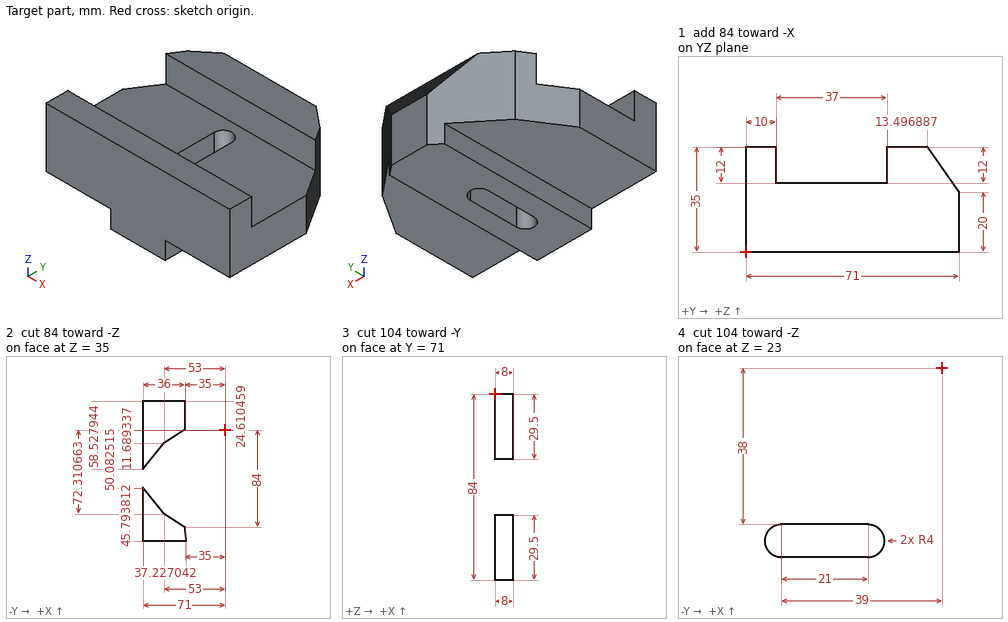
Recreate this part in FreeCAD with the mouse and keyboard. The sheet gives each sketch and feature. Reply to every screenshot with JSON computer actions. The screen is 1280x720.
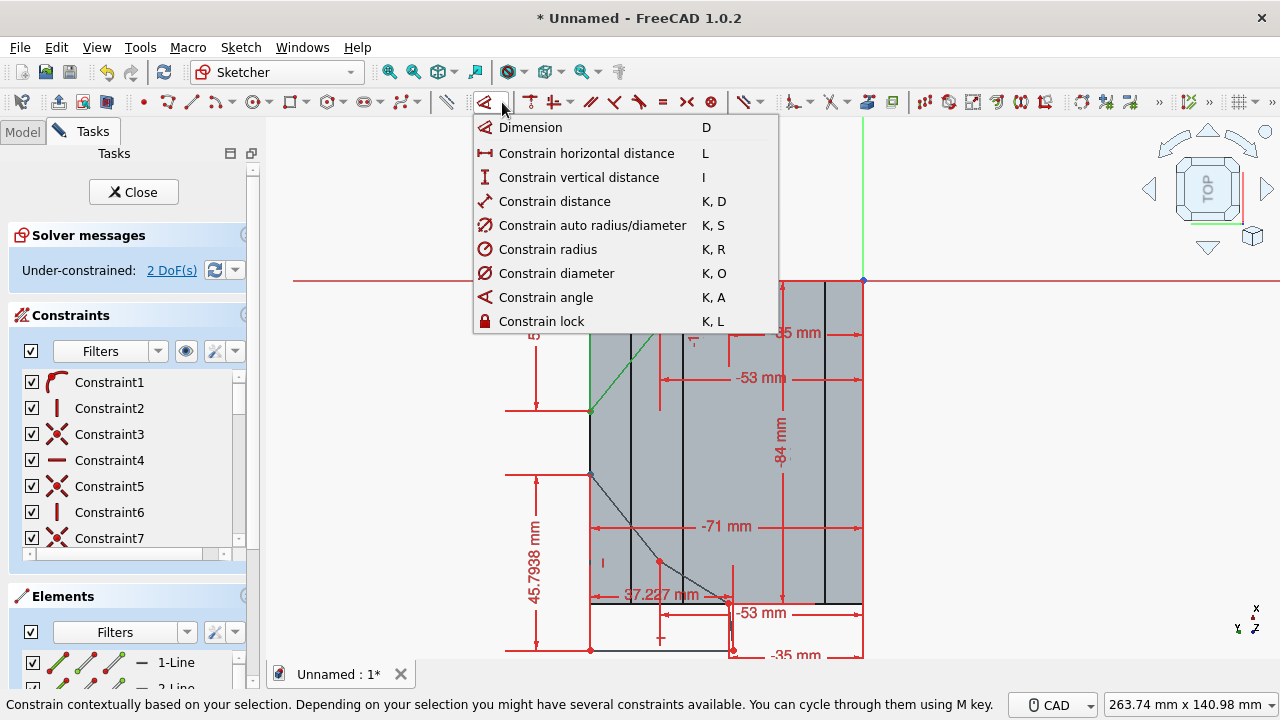
{"action": "left_click", "coordinate": [626, 177]}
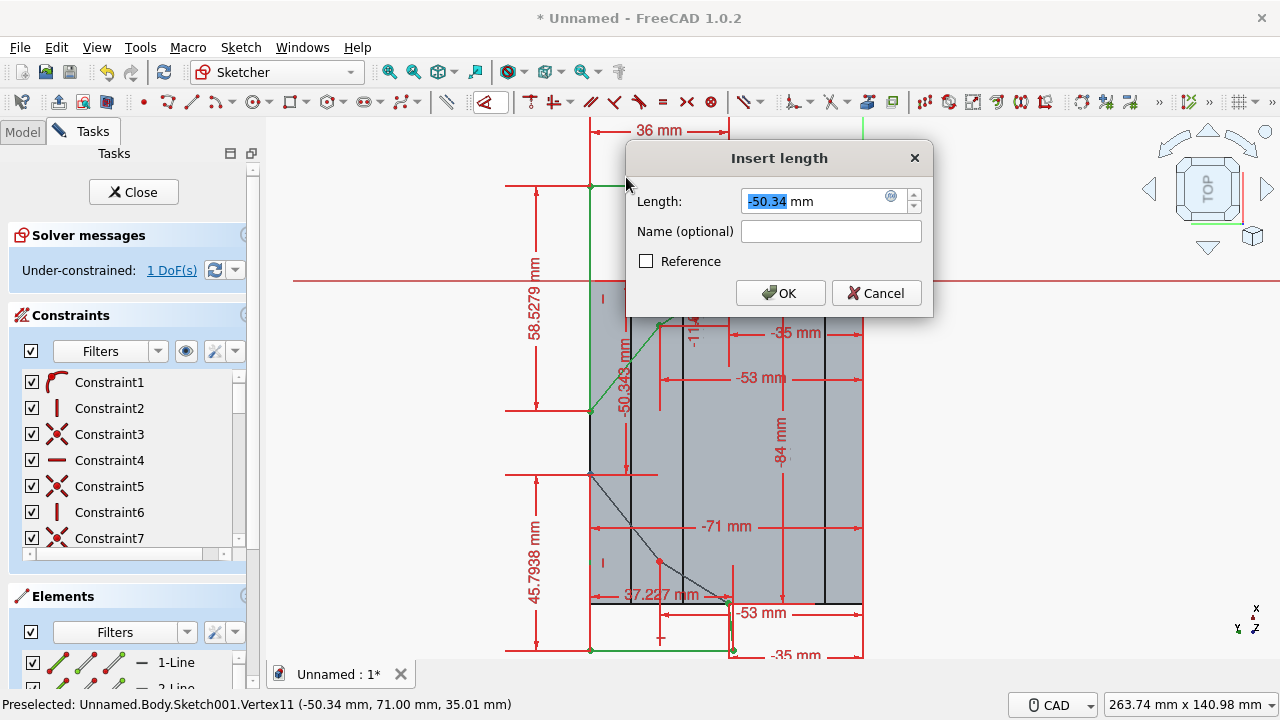
{"action": "type", "text": "-50.082515"}
{"action": "key", "text": "Return"}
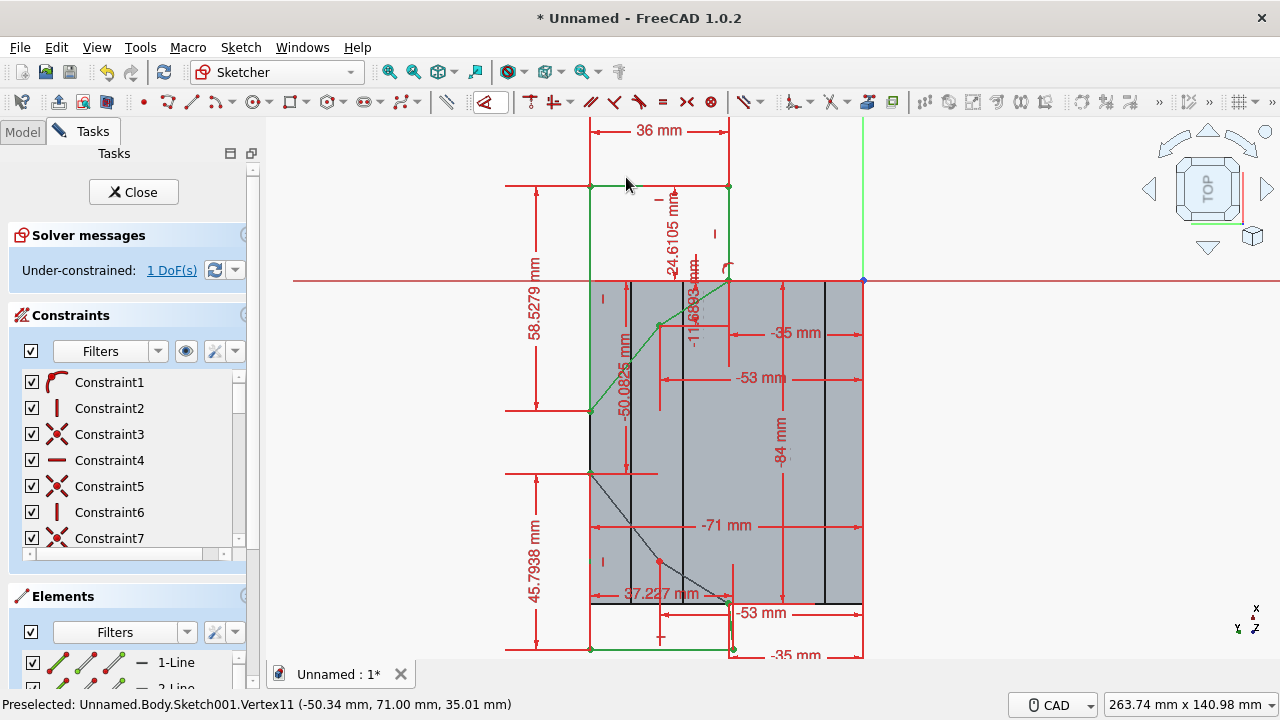
{"action": "left_click", "coordinate": [660, 561]}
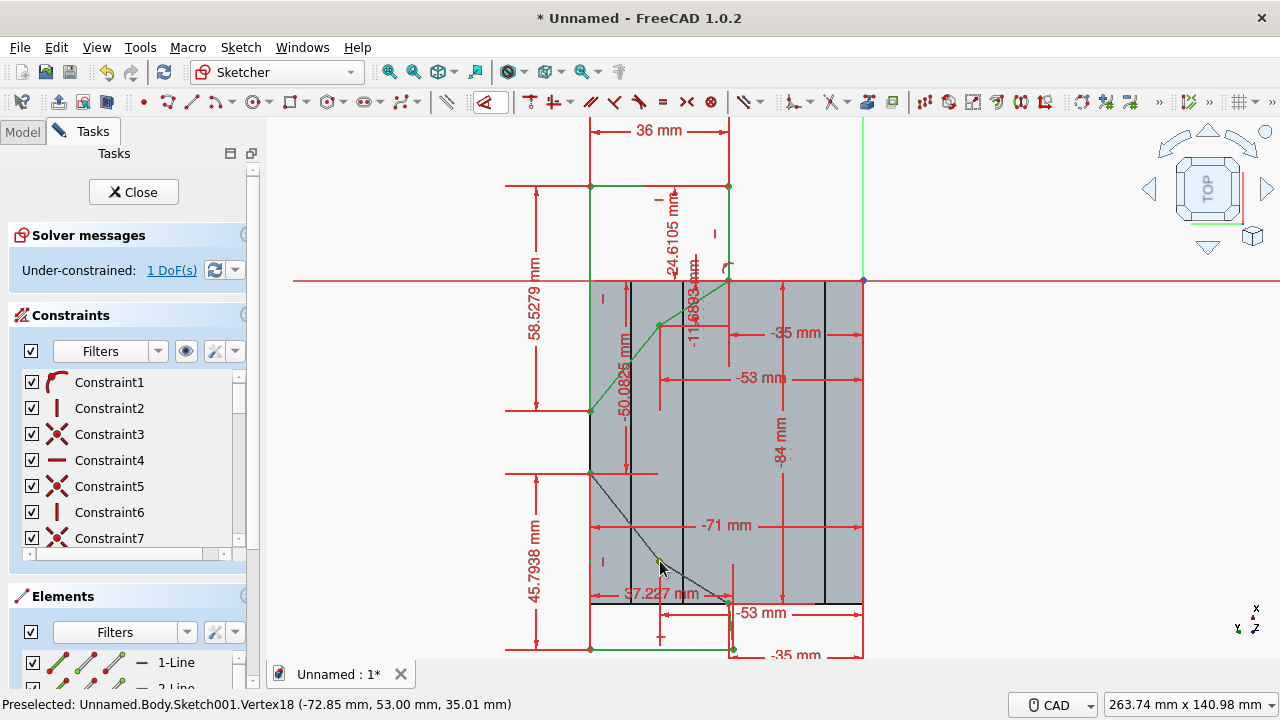
{"action": "left_click", "coordinate": [502, 102]}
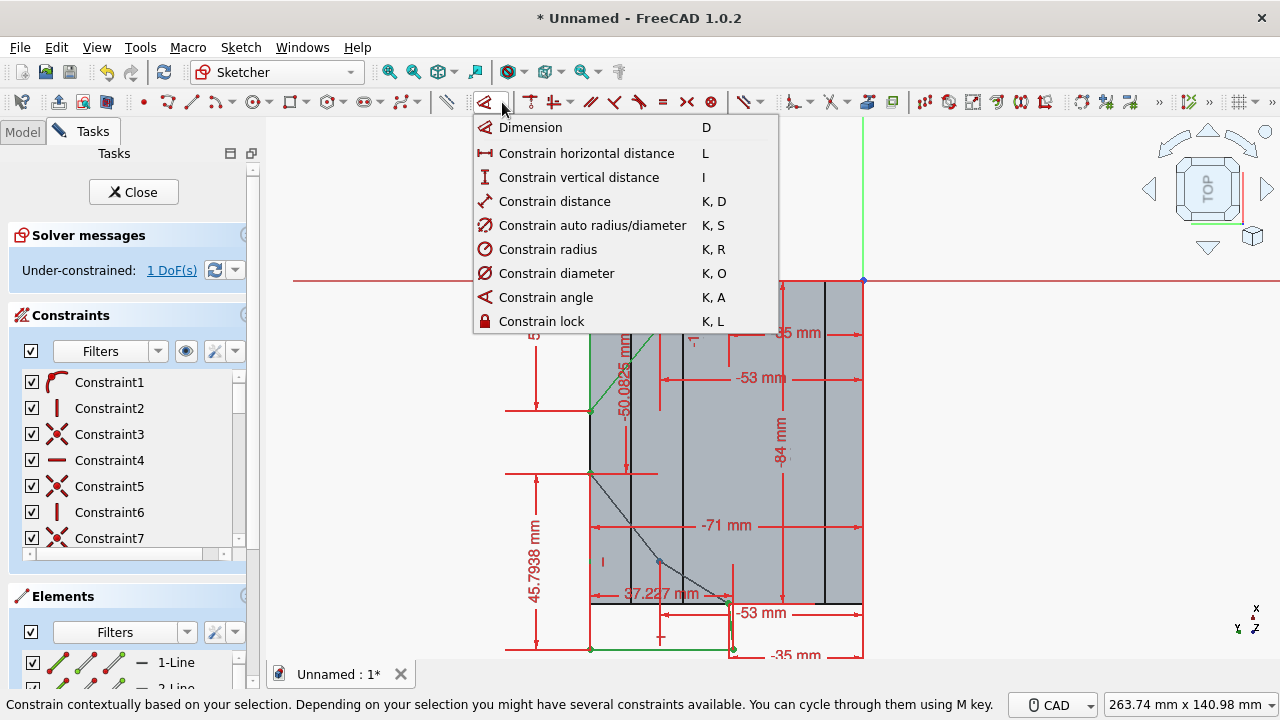
{"action": "left_click", "coordinate": [626, 177]}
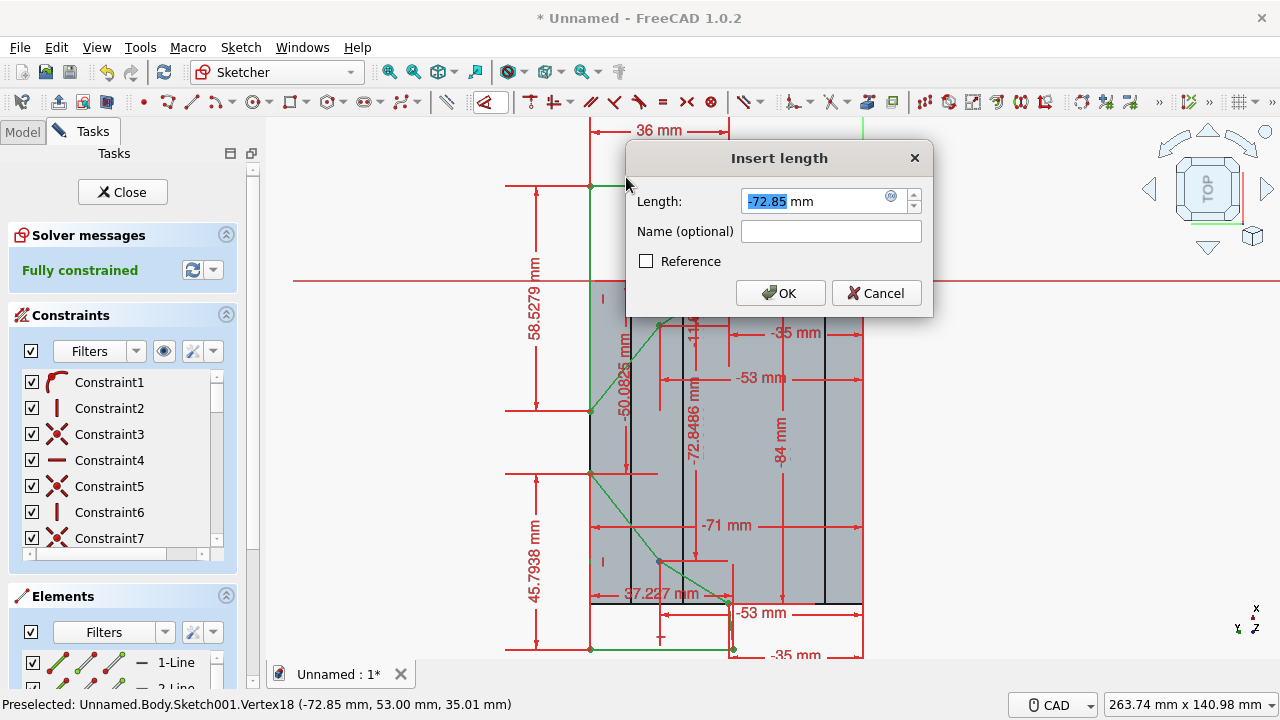
{"action": "type", "text": "-72.310663"}
{"action": "key", "text": "Return"}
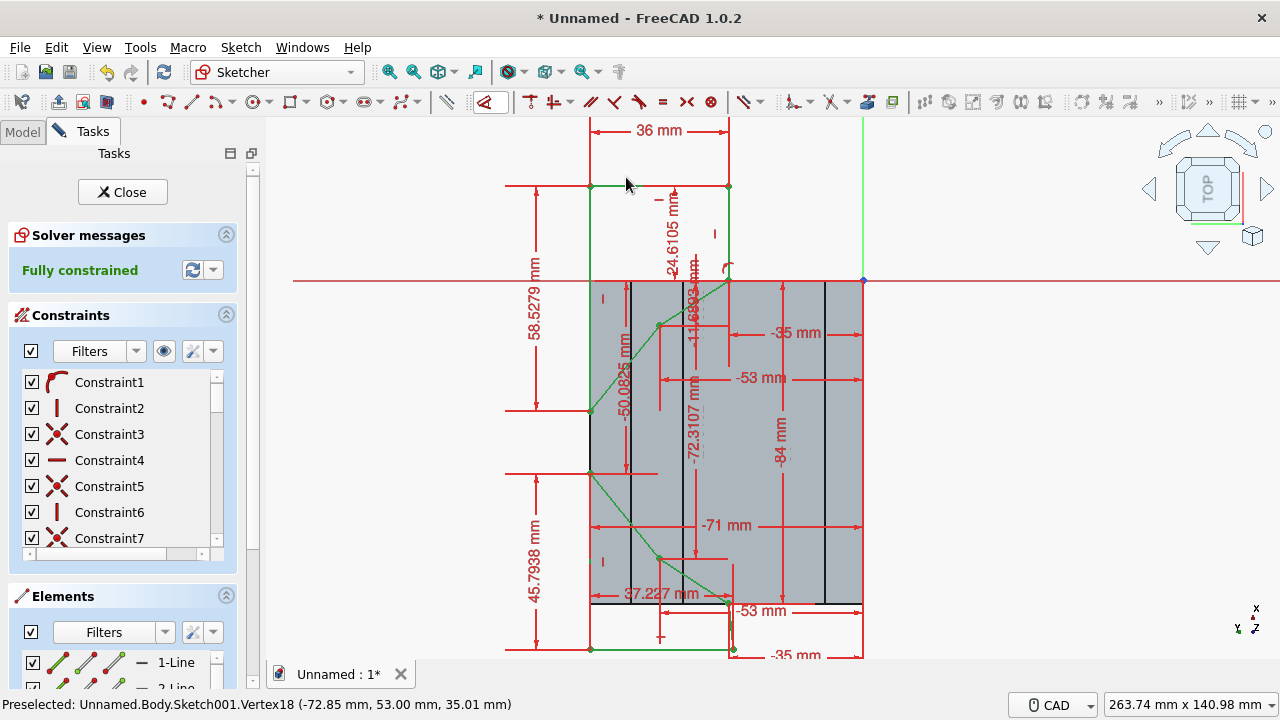
{"action": "left_click", "coordinate": [123, 192]}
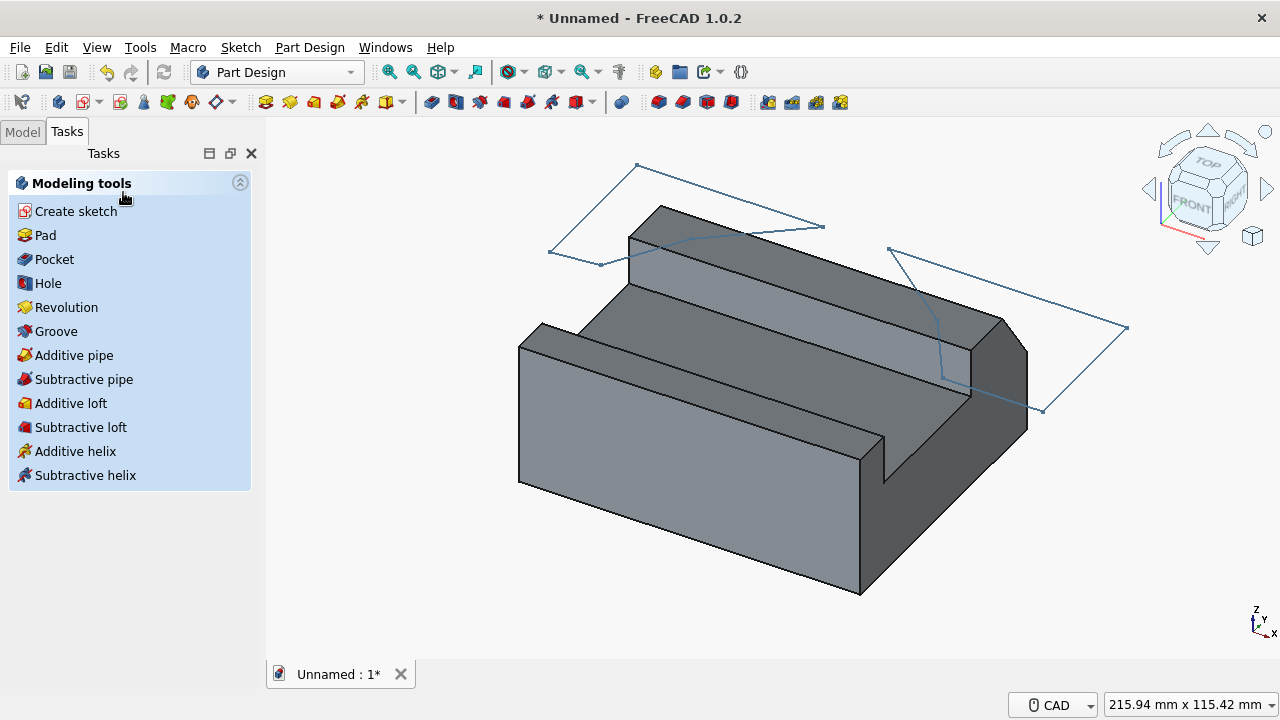
{"action": "left_click", "coordinate": [432, 102]}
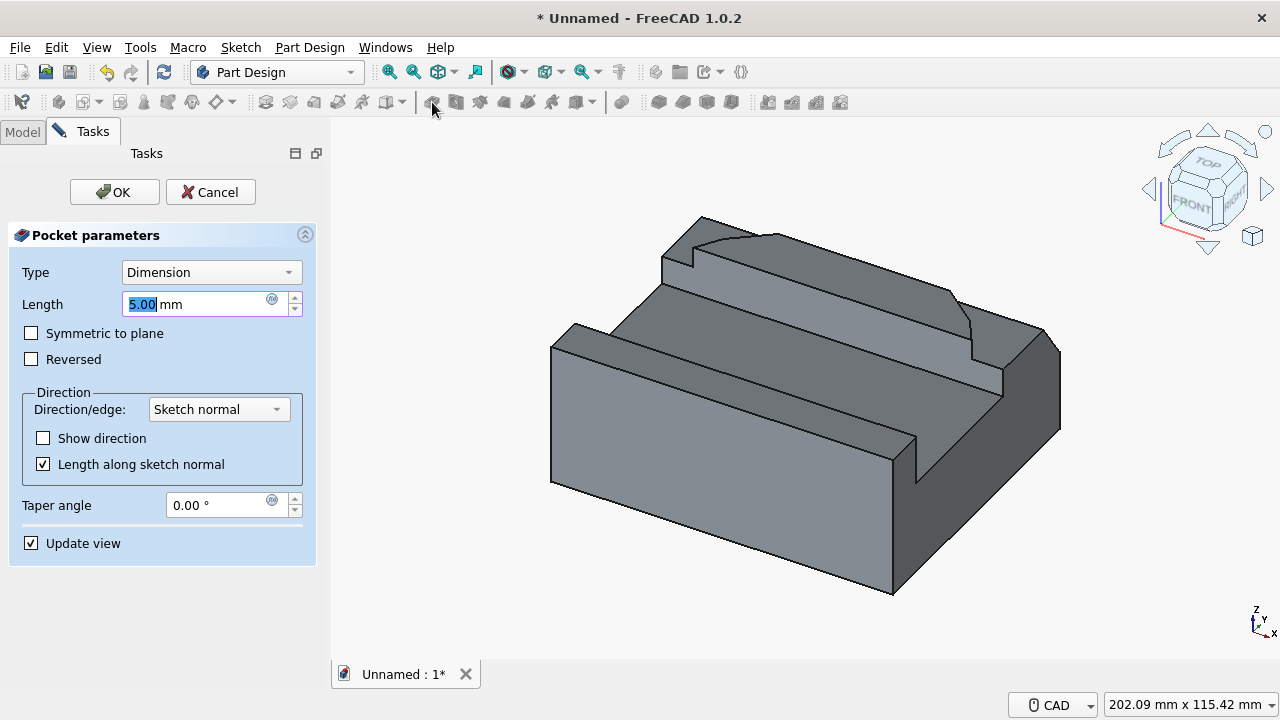
{"action": "type", "text": "84"}
{"action": "key", "text": "Tab"}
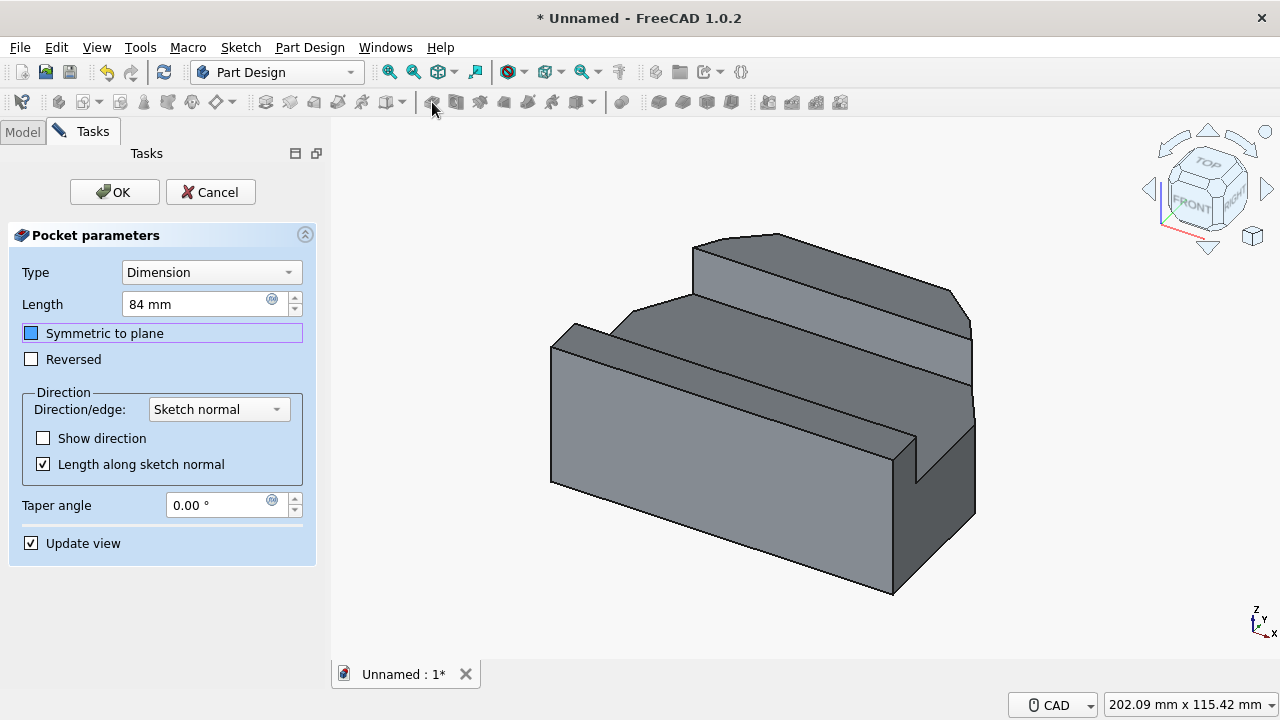
{"action": "left_click", "coordinate": [115, 192]}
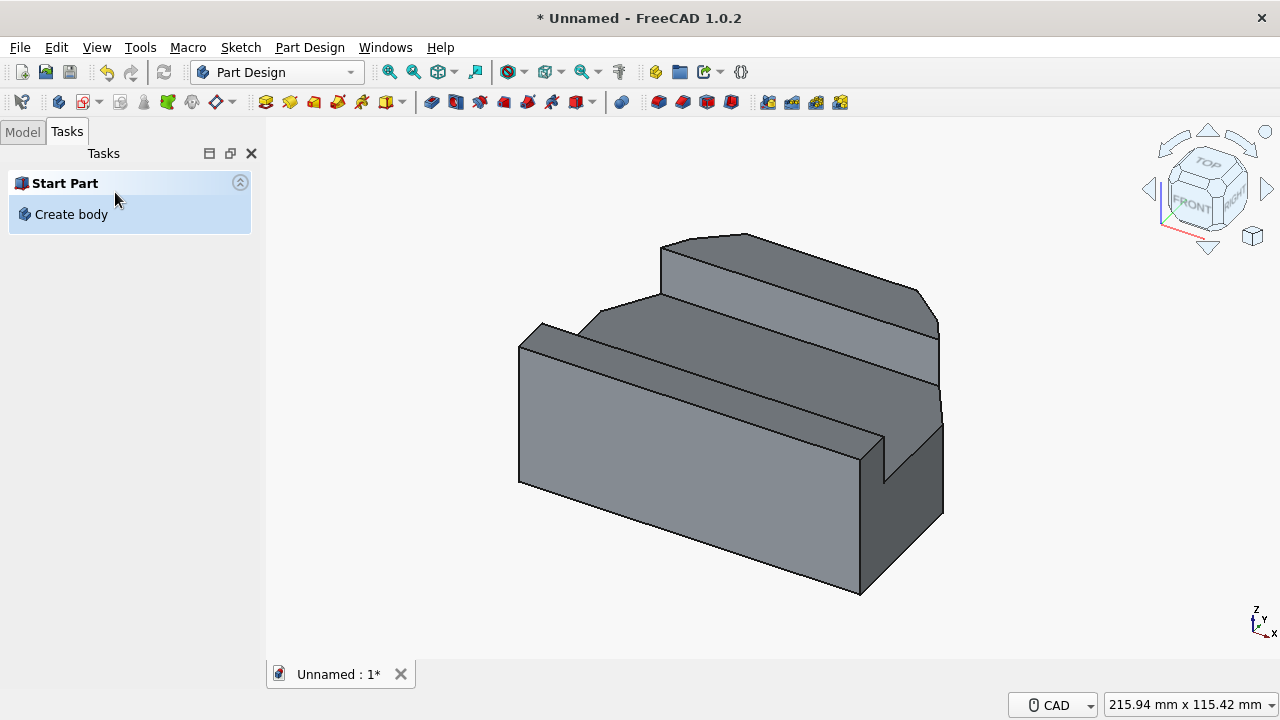
{"action": "key", "text": "4"}